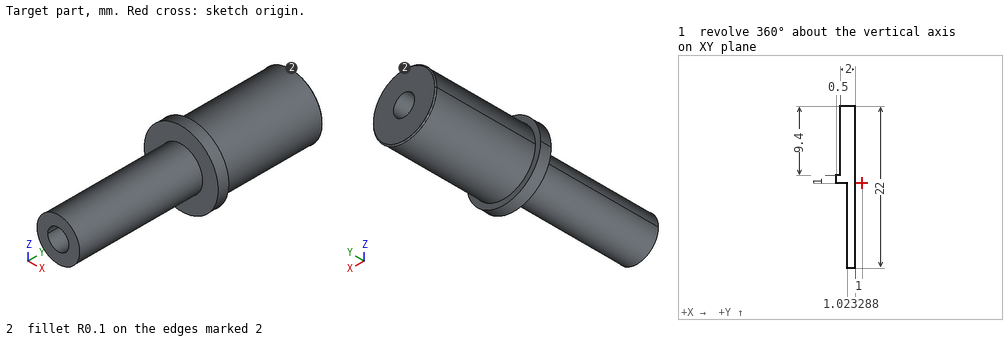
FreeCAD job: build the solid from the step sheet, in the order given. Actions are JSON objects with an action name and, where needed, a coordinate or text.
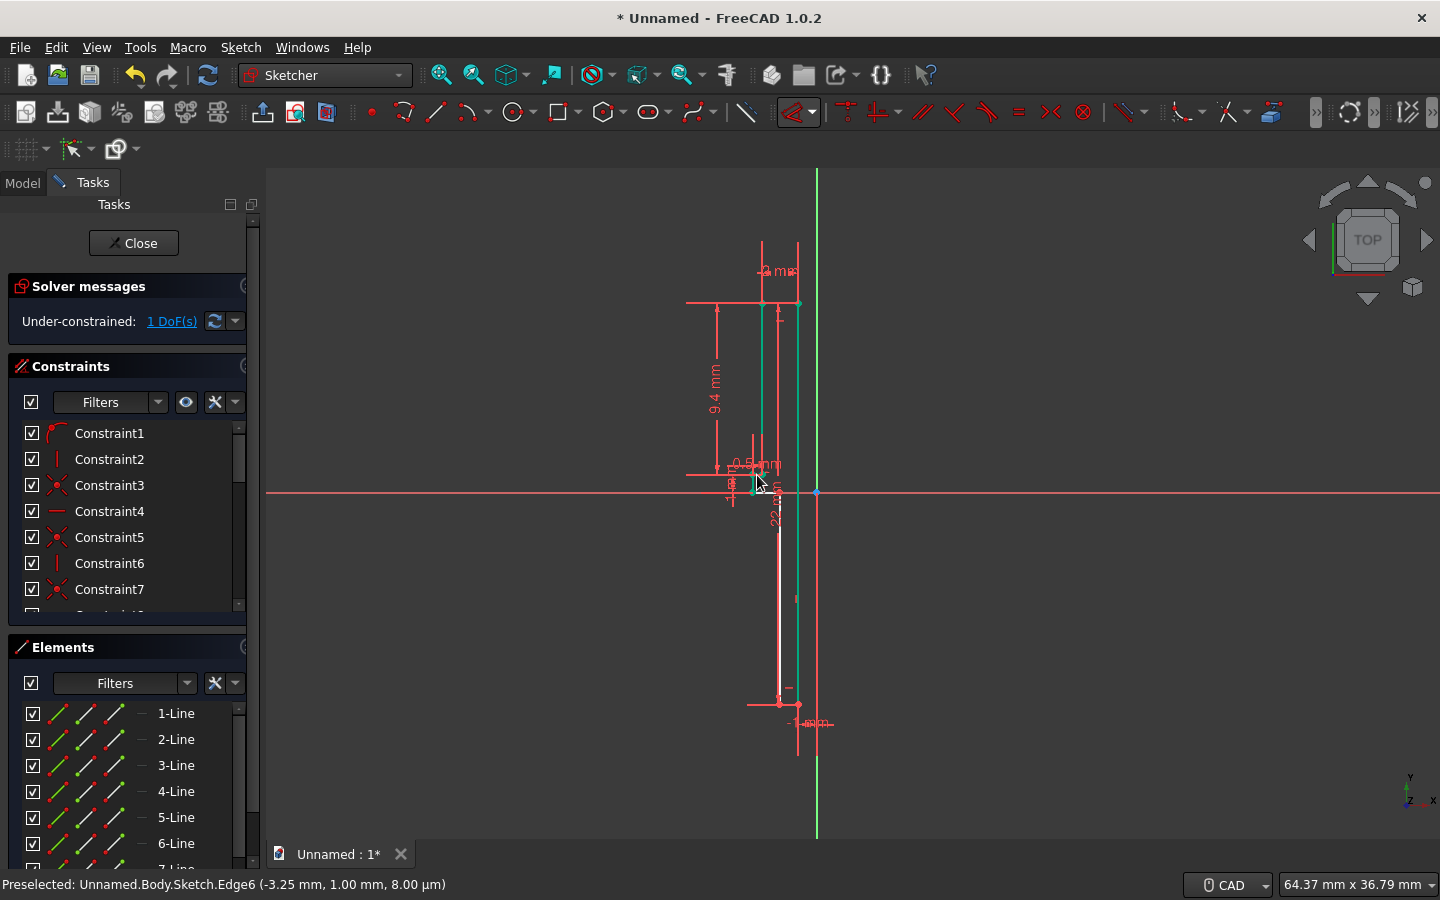
{"action": "scroll", "coordinate": [785, 705], "scroll_direction": "up", "scroll_amount": 5}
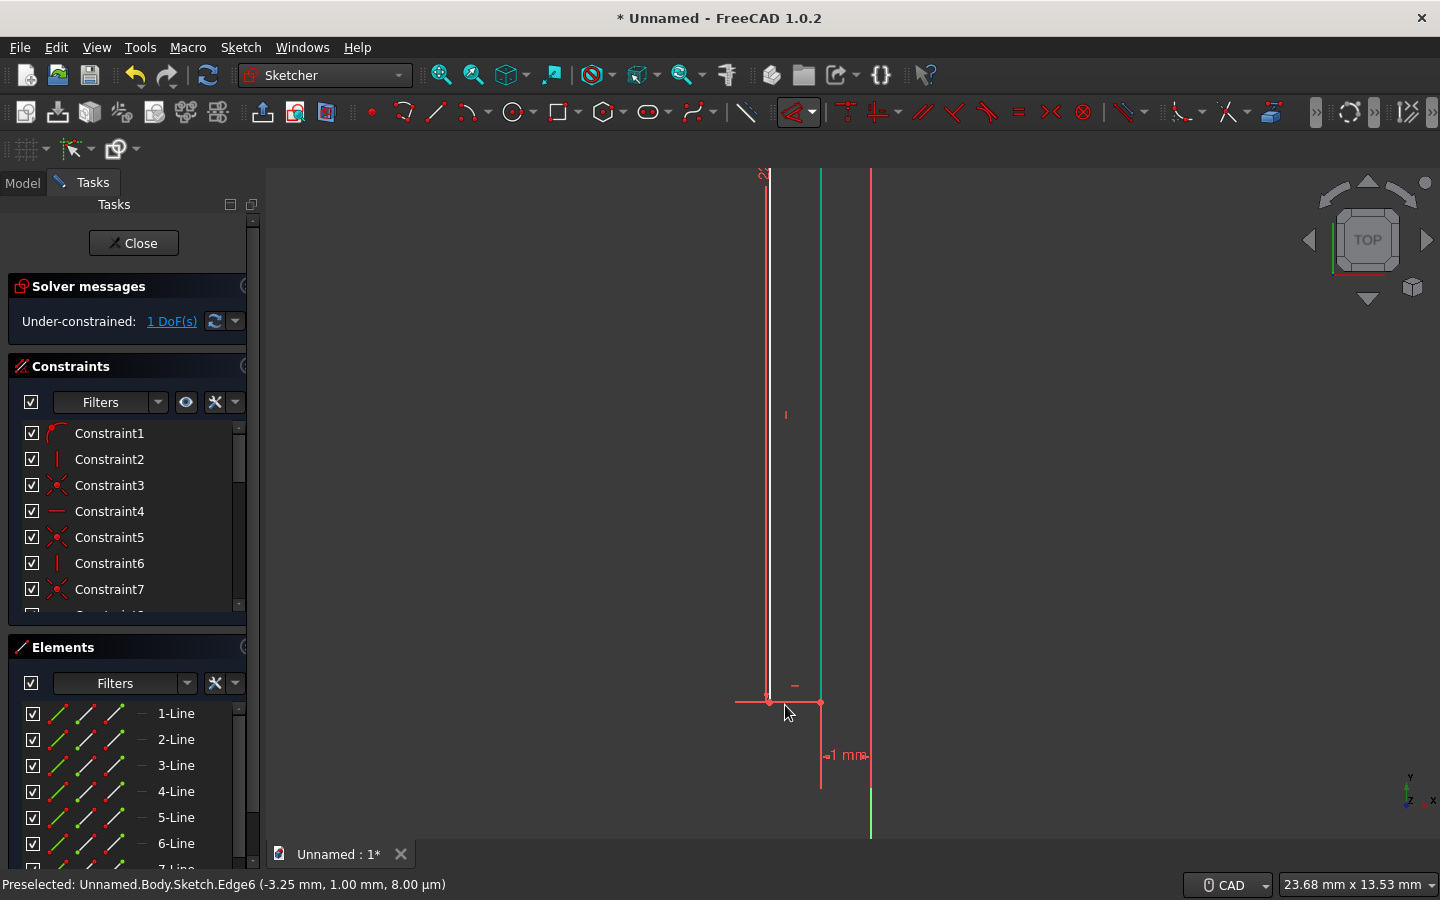
{"action": "left_click", "coordinate": [785, 702]}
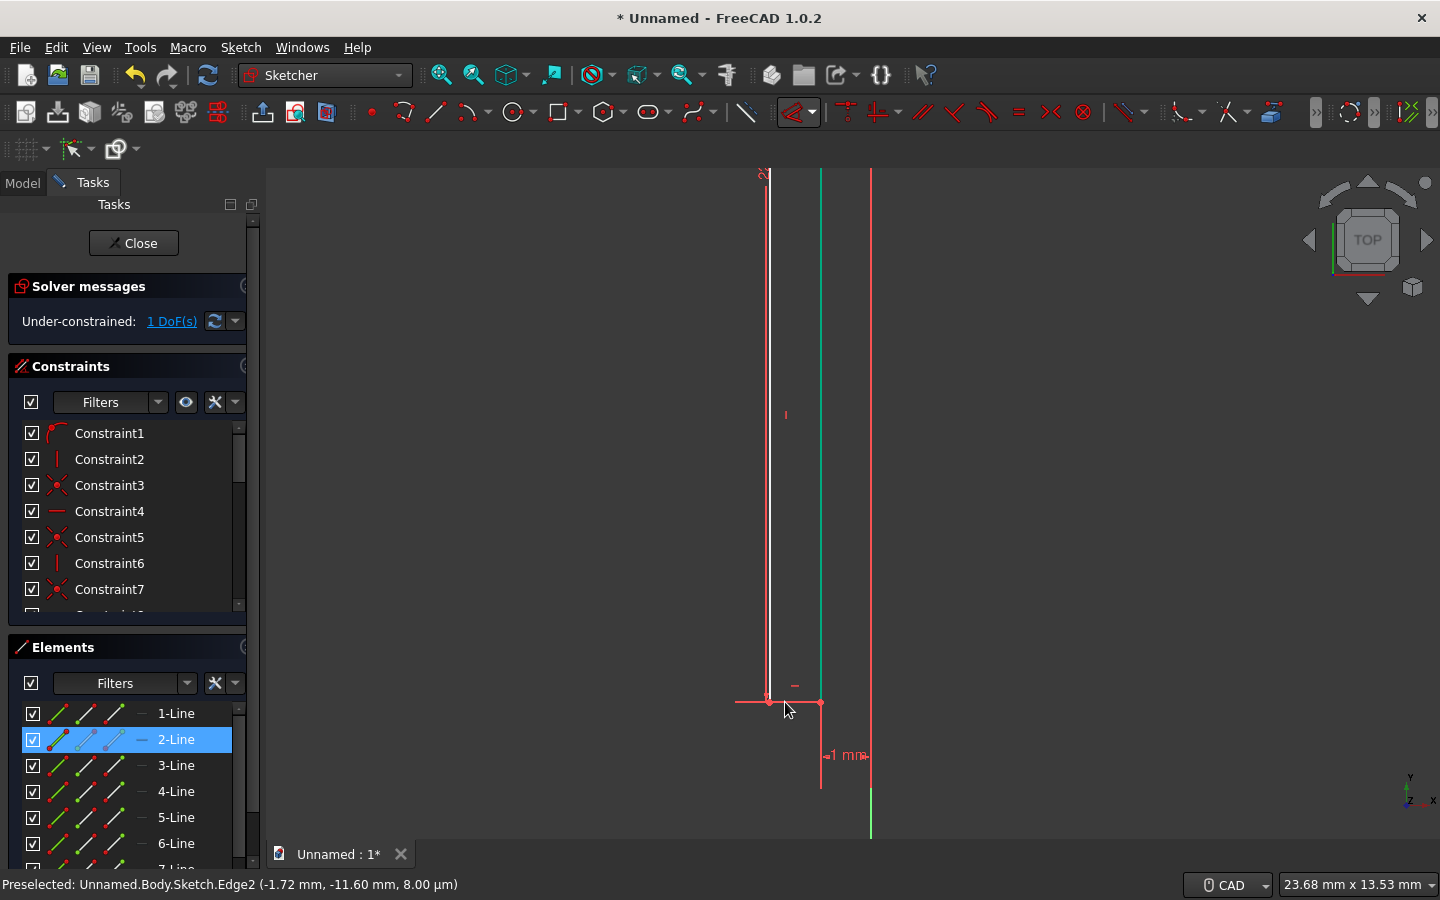
{"action": "left_click", "coordinate": [814, 112]}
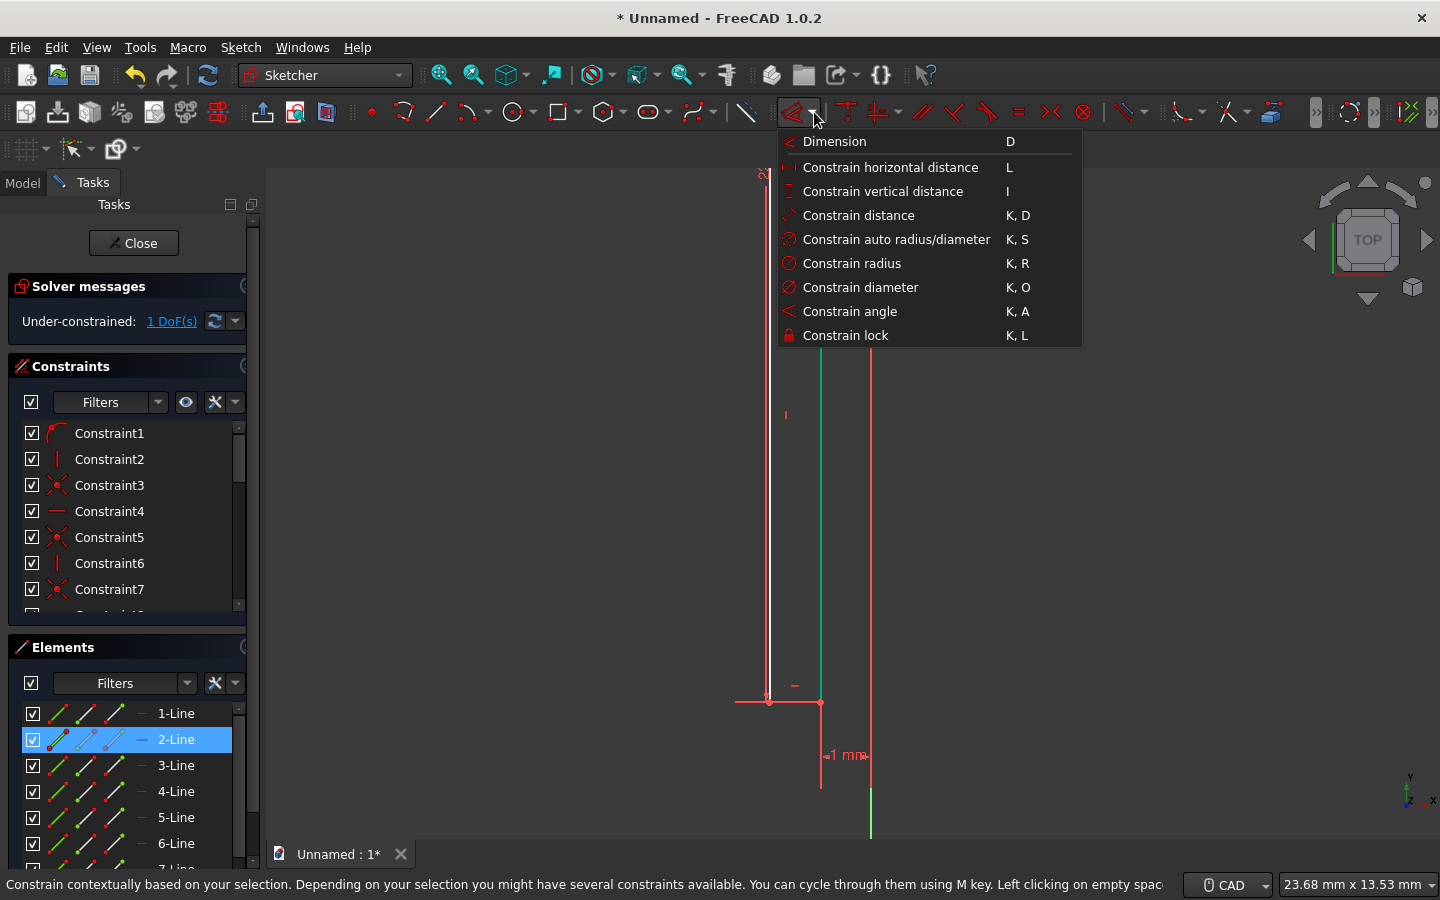
{"action": "left_click", "coordinate": [930, 167]}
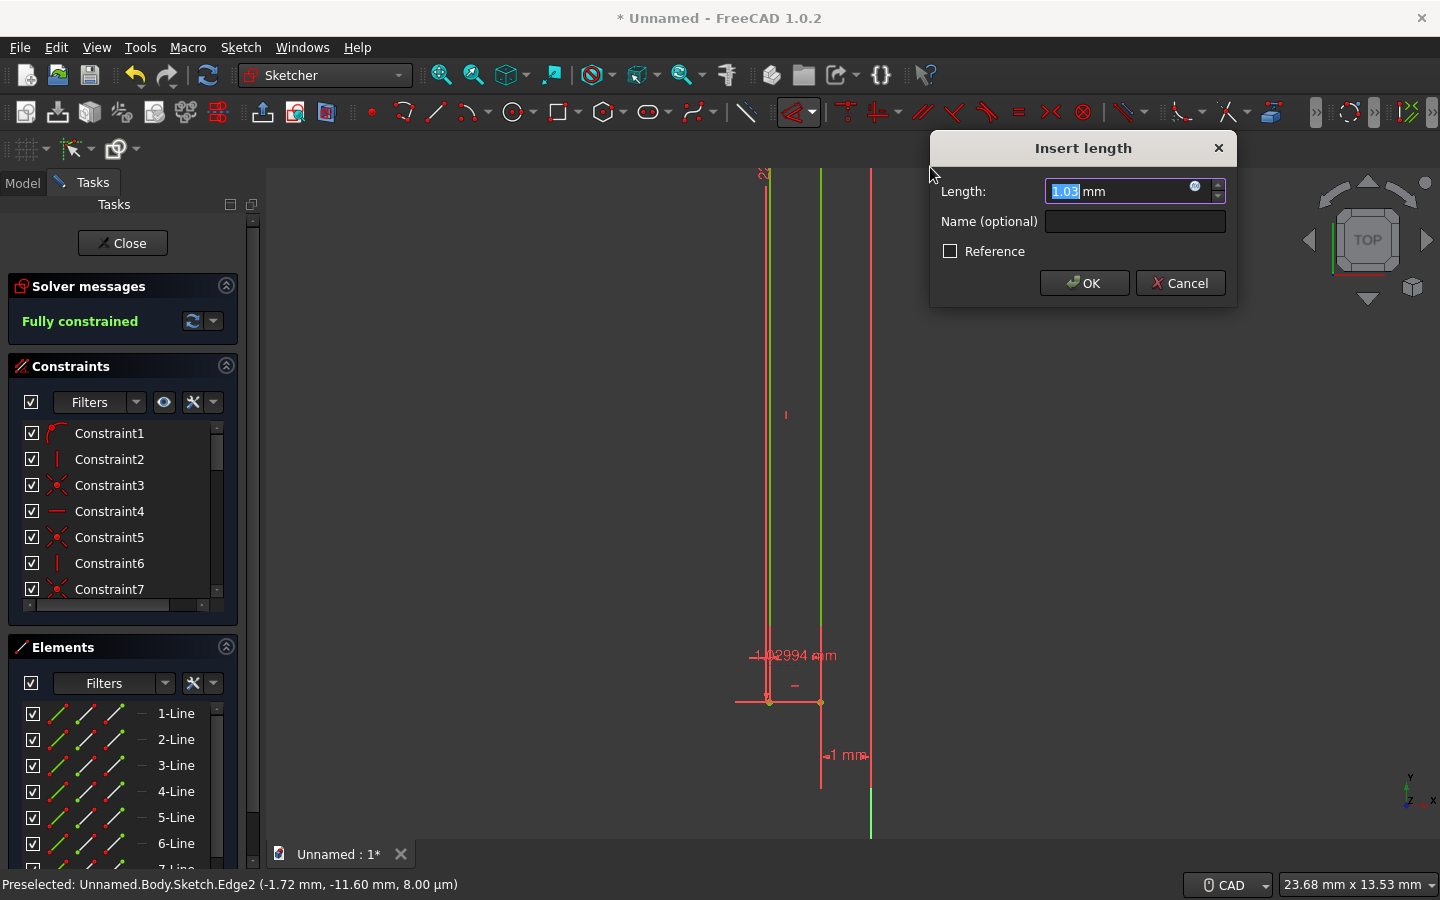
{"action": "type", "text": "1.023288"}
{"action": "key", "text": "Return"}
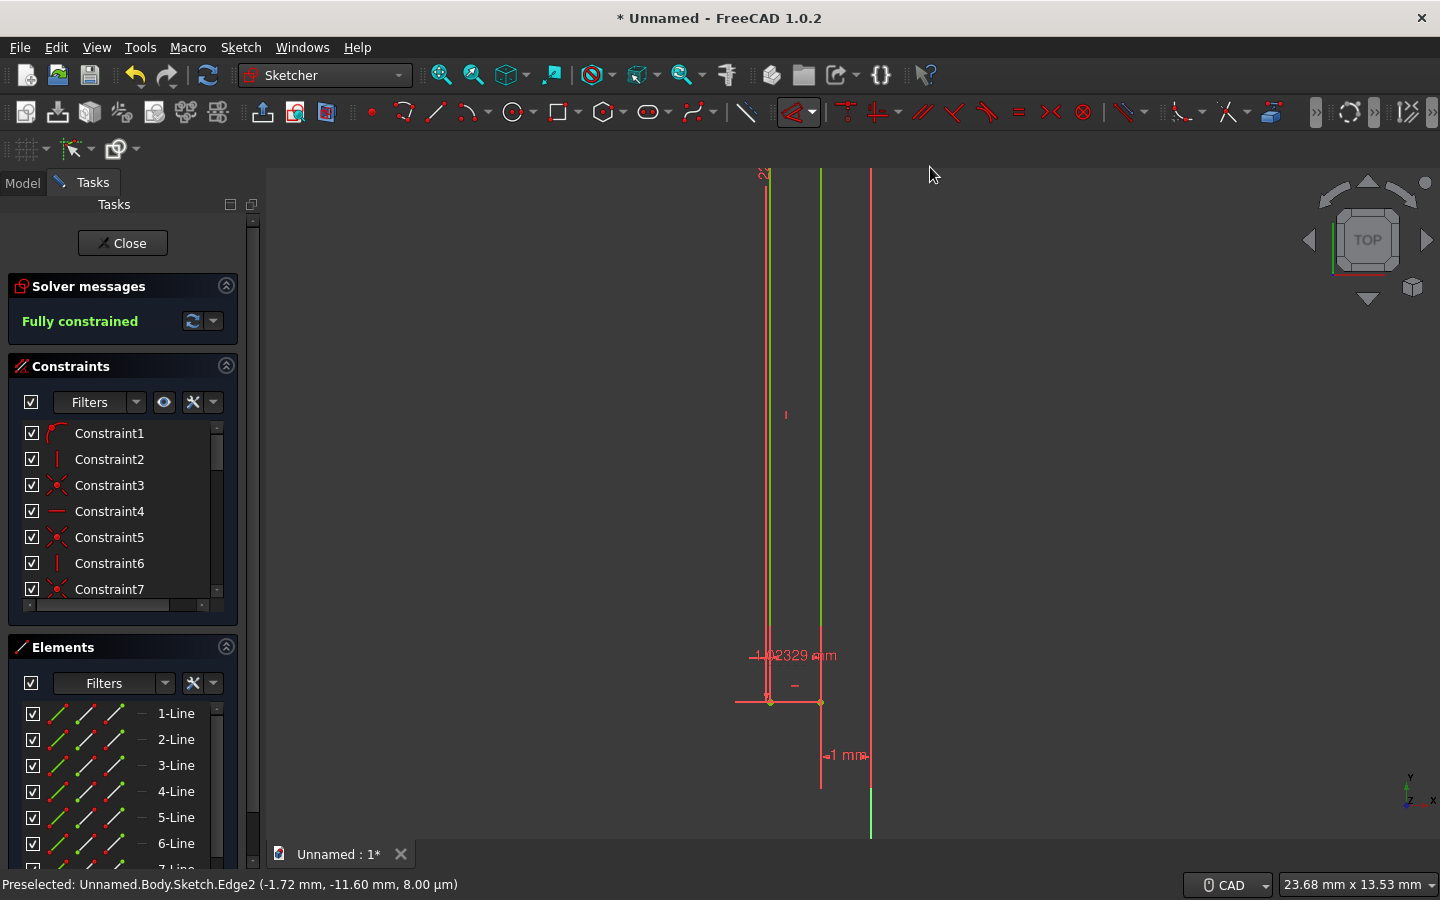
{"action": "left_click", "coordinate": [123, 243]}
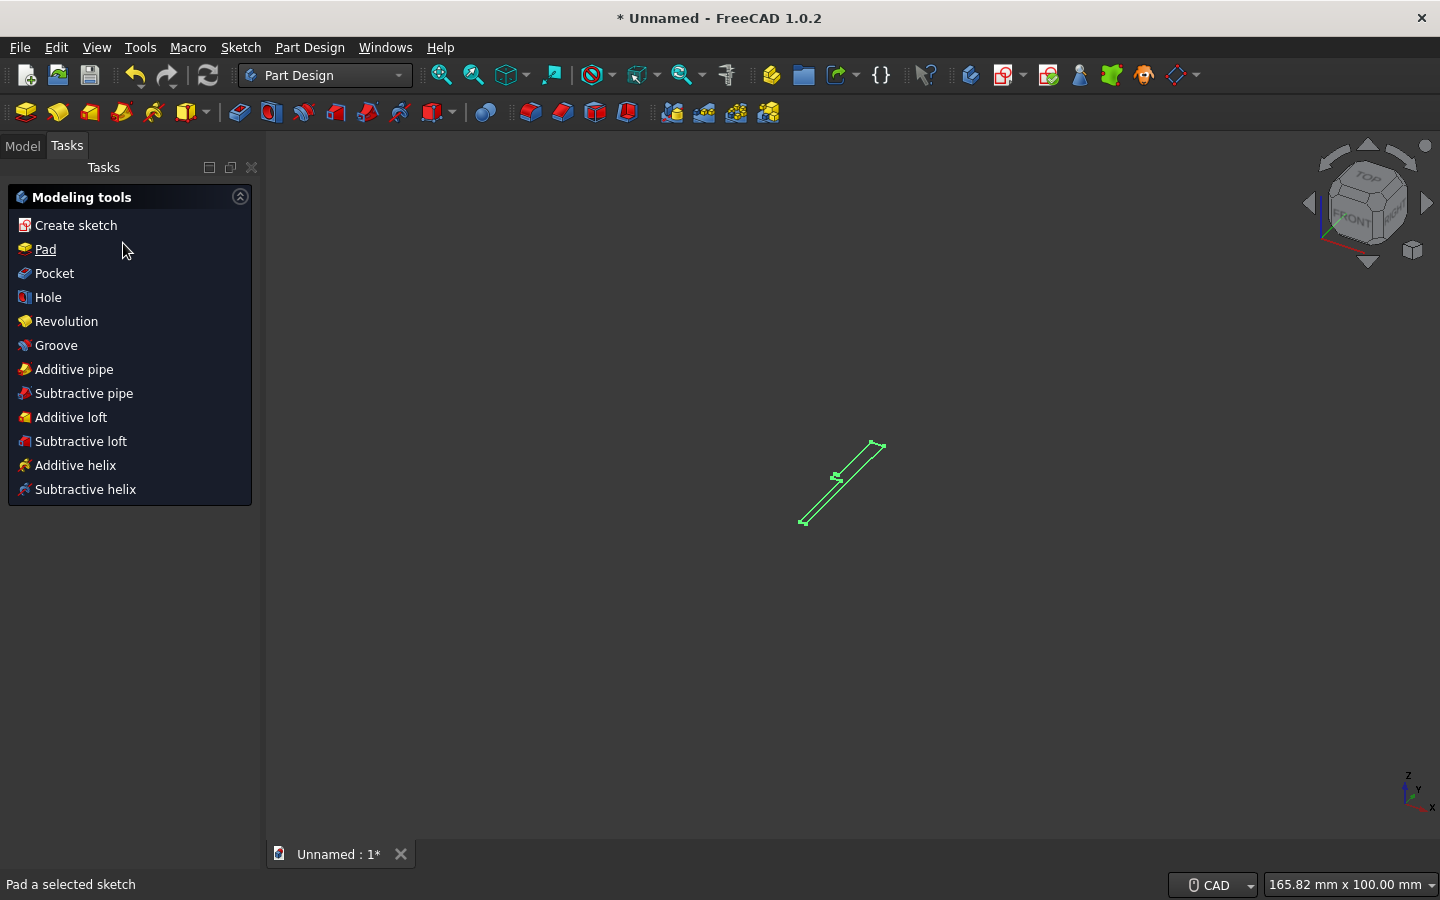
{"action": "left_click", "coordinate": [58, 112]}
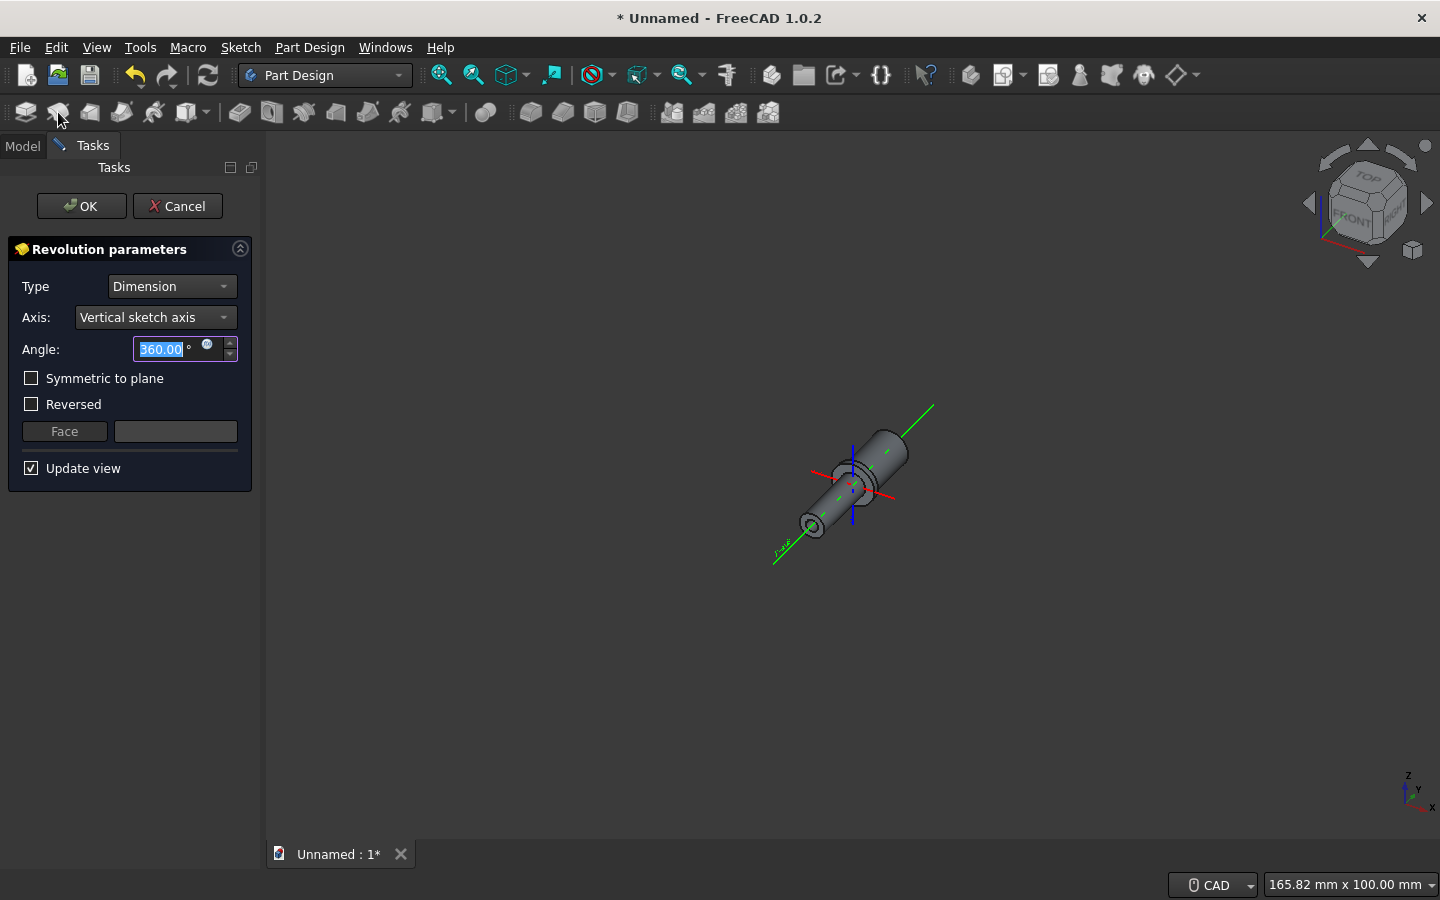
{"action": "left_click", "coordinate": [82, 206]}